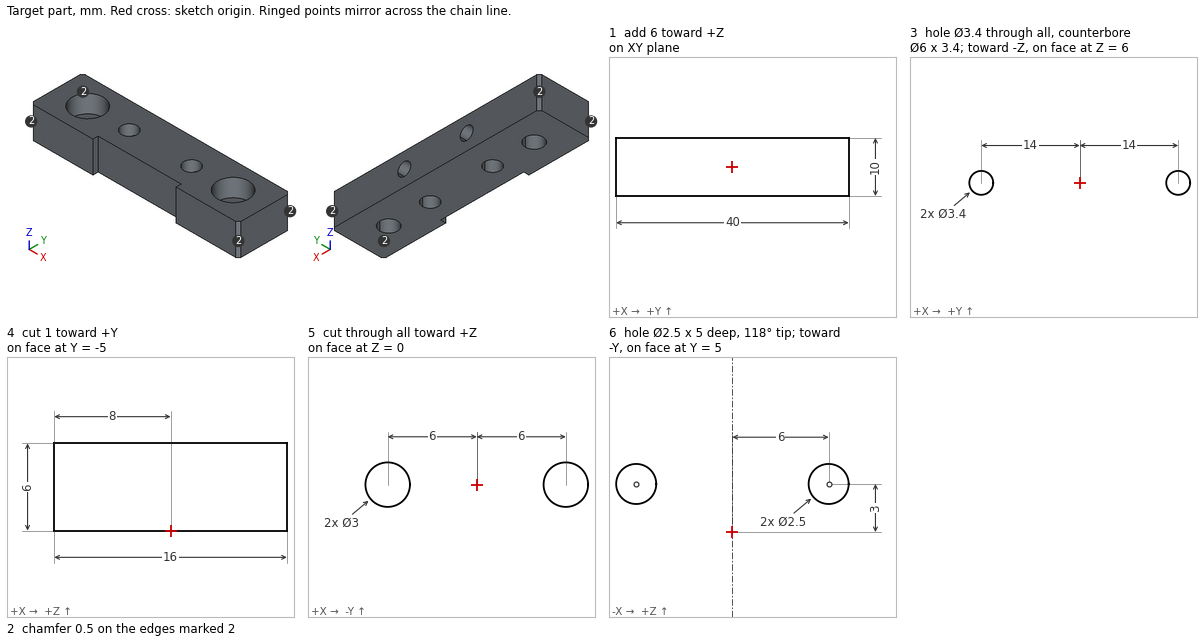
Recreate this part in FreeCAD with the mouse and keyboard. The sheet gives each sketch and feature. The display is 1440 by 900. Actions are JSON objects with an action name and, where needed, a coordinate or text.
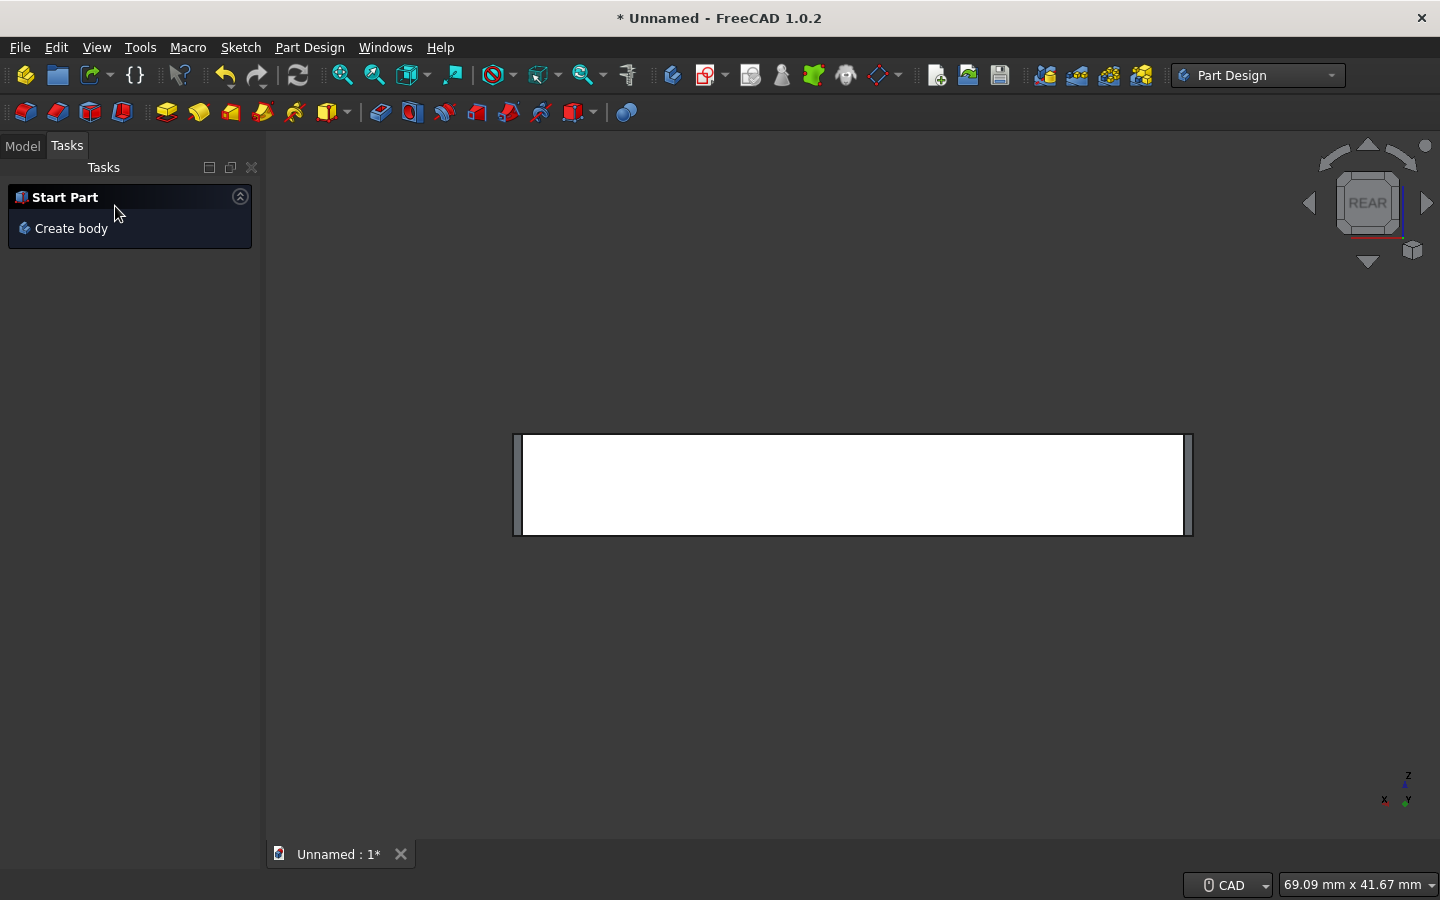
{"action": "left_click", "coordinate": [664, 484]}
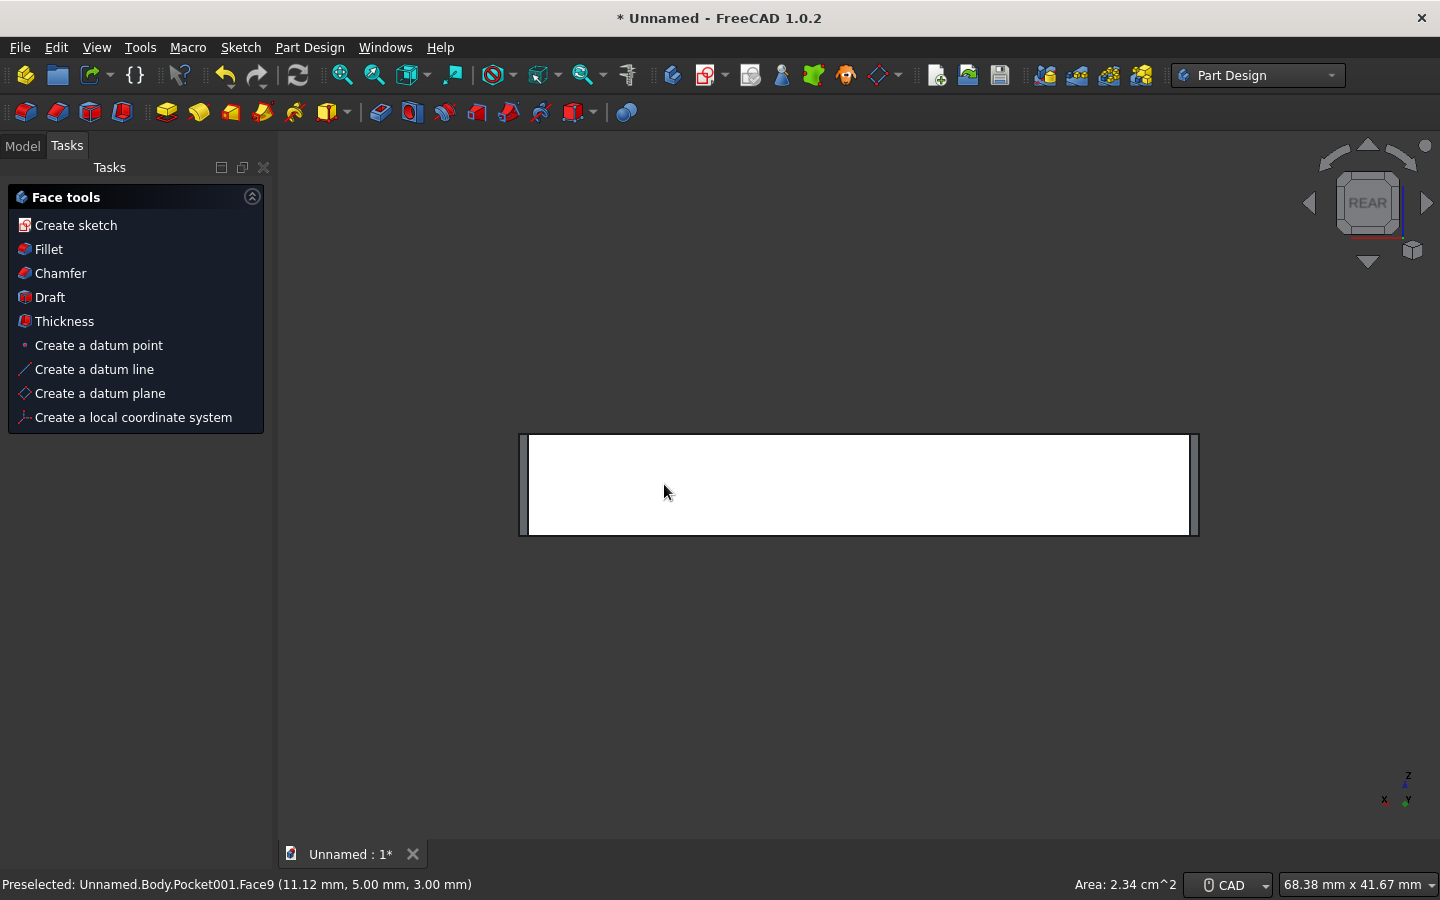
{"action": "left_click", "coordinate": [706, 76]}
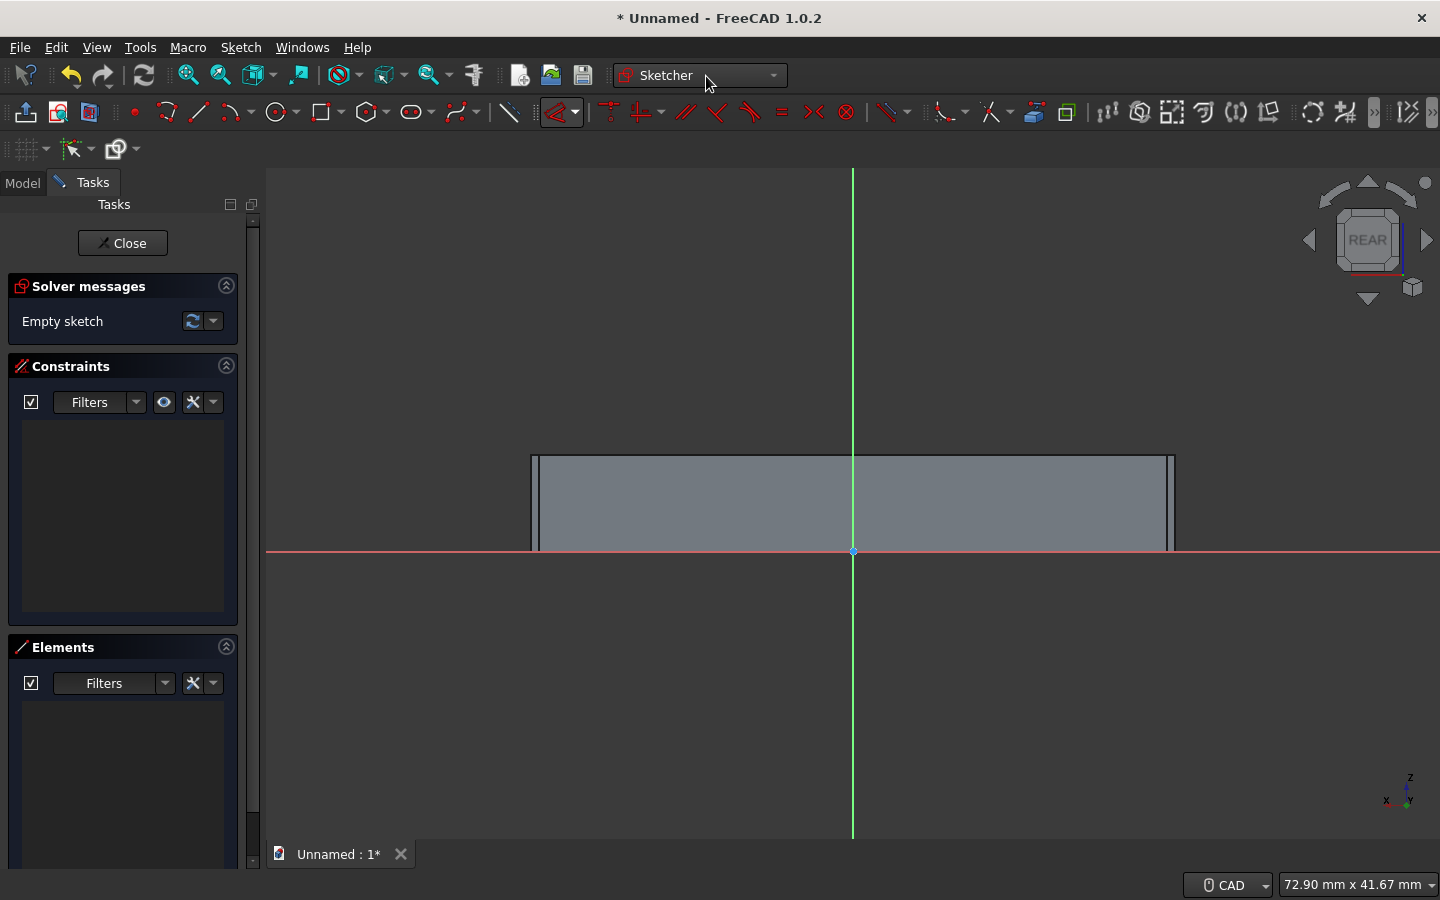
{"action": "scroll", "coordinate": [893, 526], "scroll_direction": "up", "scroll_amount": 5}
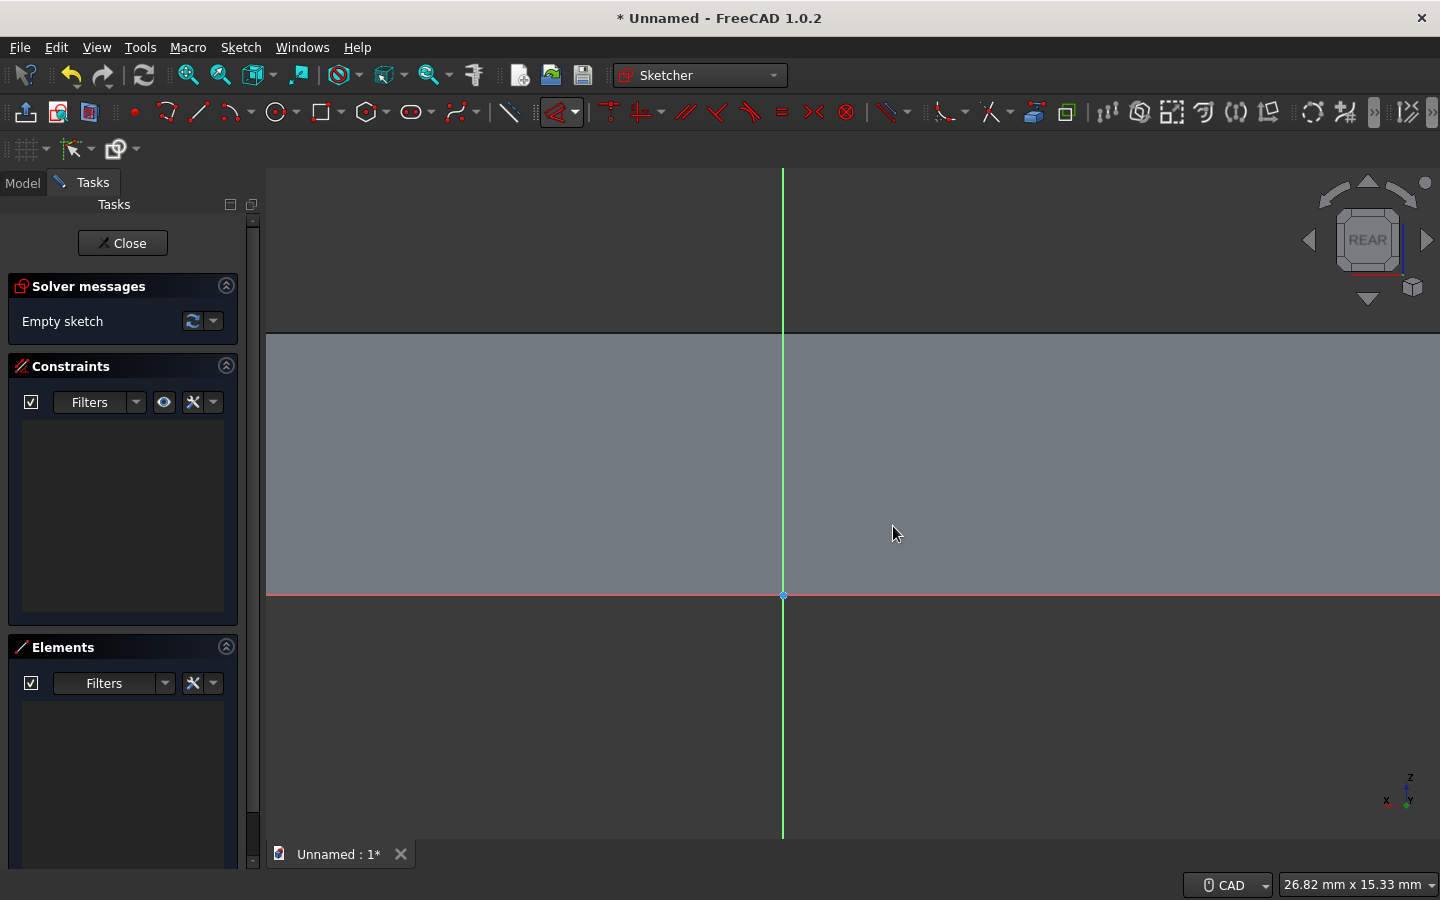
{"action": "left_click", "coordinate": [276, 112]}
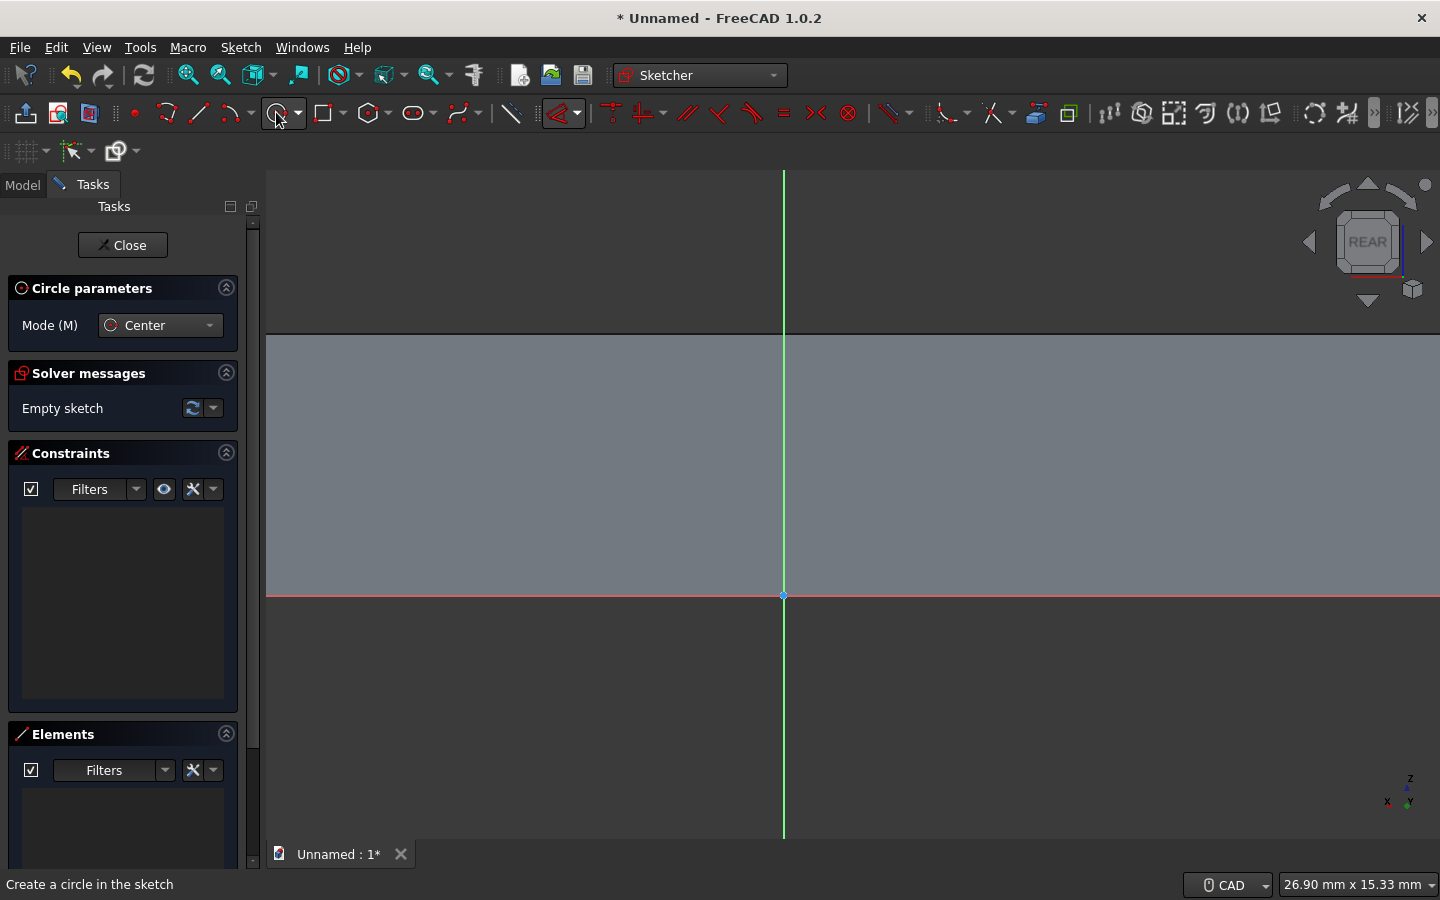
{"action": "left_click", "coordinate": [1045, 465]}
{"action": "mouse_move", "coordinate": [1084, 426]}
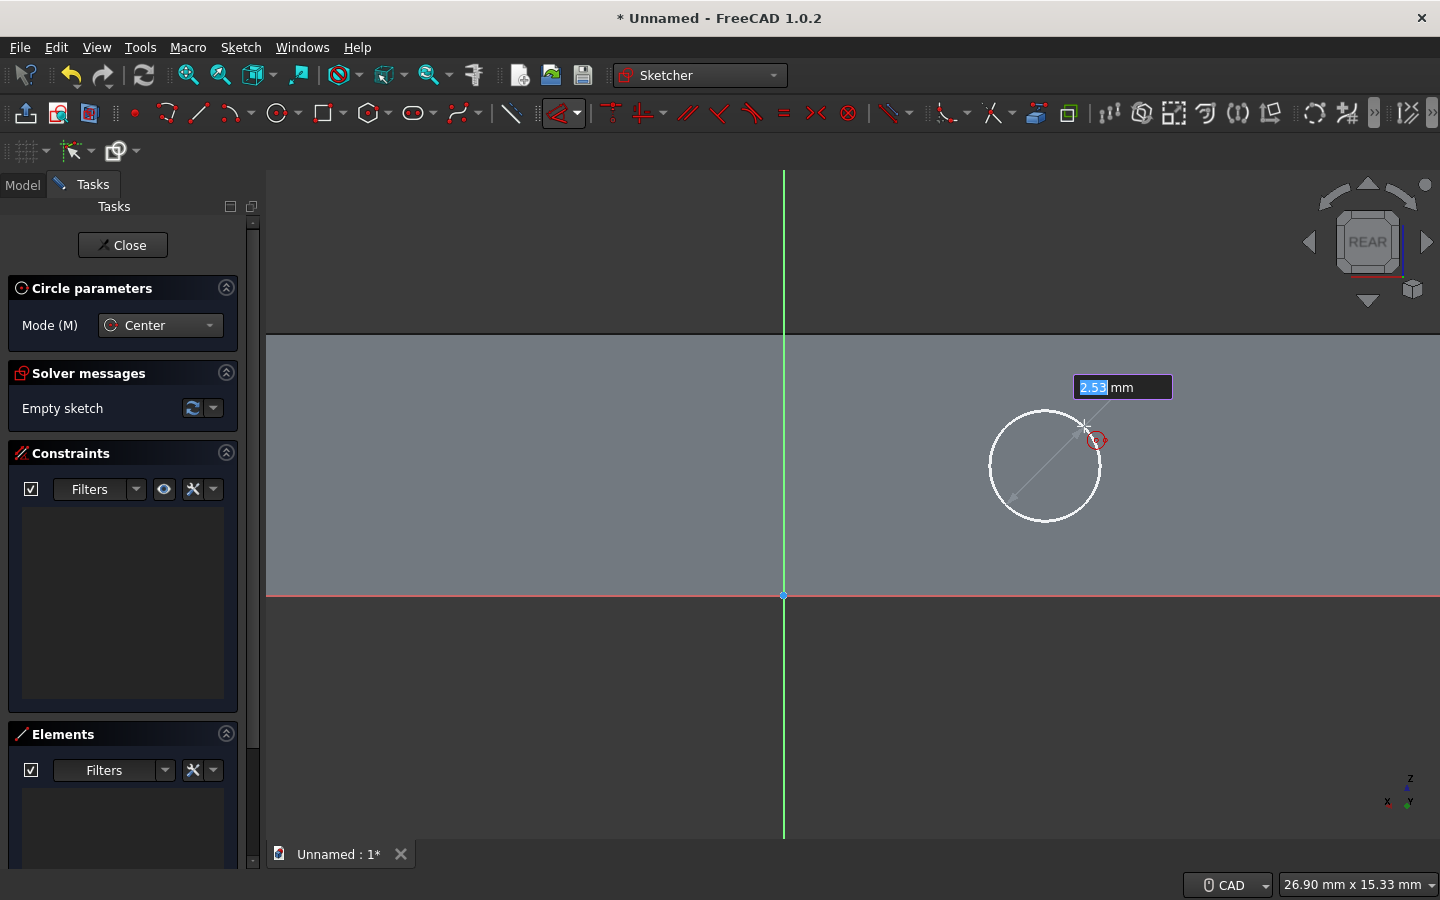
{"action": "type", "text": "2.5"}
{"action": "key", "text": "Return"}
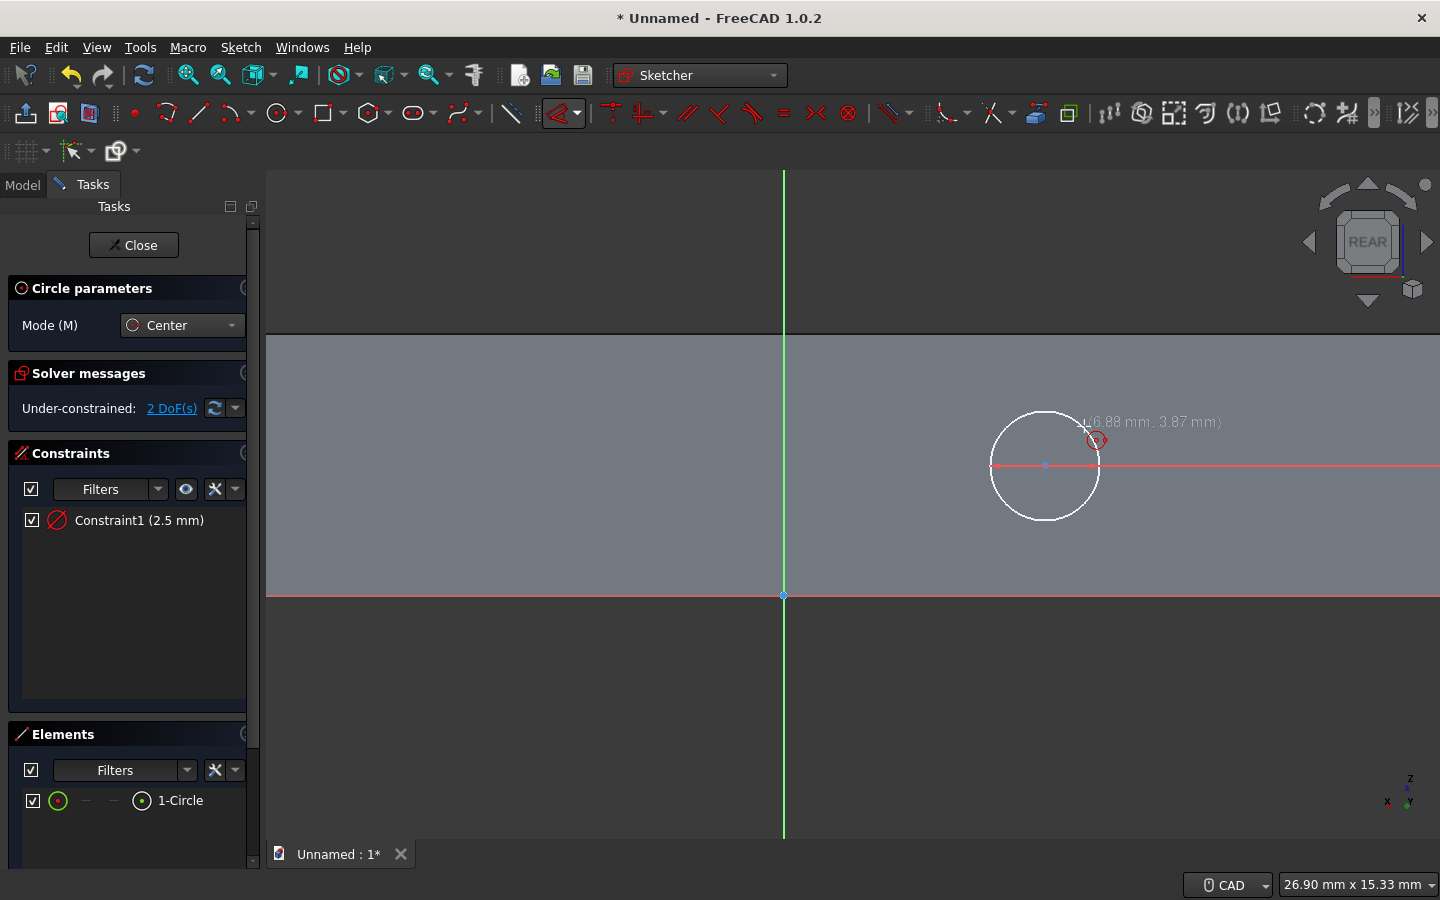
{"action": "left_click", "coordinate": [522, 465]}
{"action": "mouse_move", "coordinate": [560, 426]}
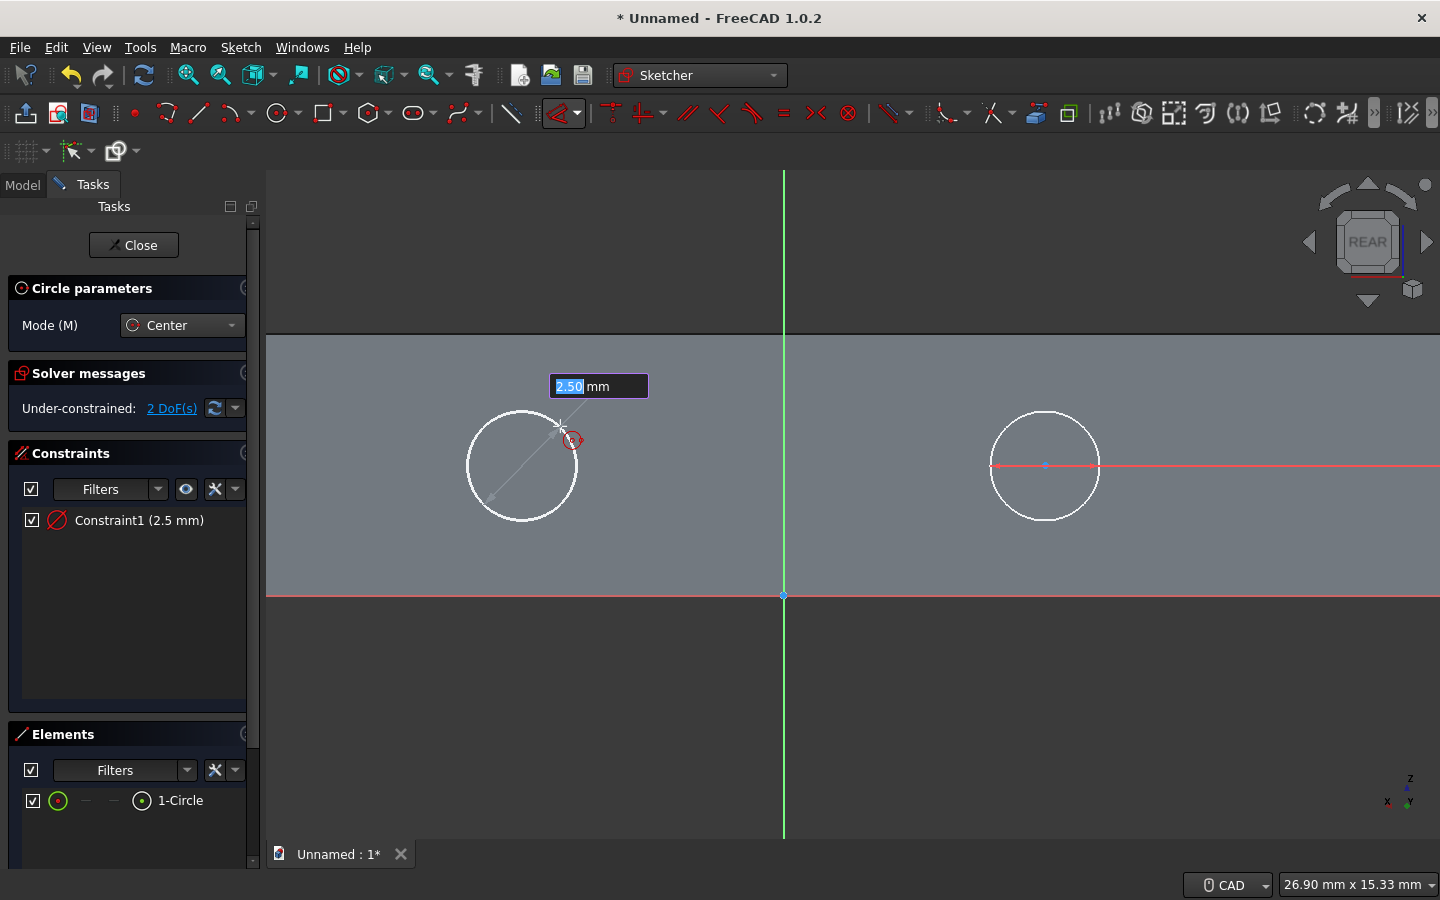
{"action": "type", "text": "2.5"}
{"action": "key", "text": "Return"}
{"action": "key", "text": "Escape"}